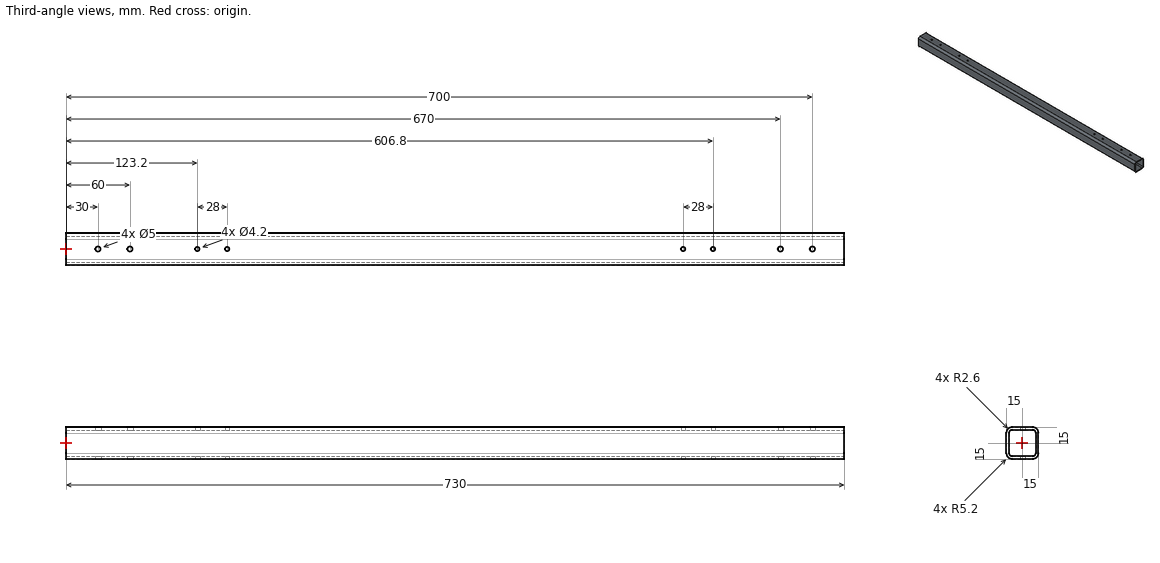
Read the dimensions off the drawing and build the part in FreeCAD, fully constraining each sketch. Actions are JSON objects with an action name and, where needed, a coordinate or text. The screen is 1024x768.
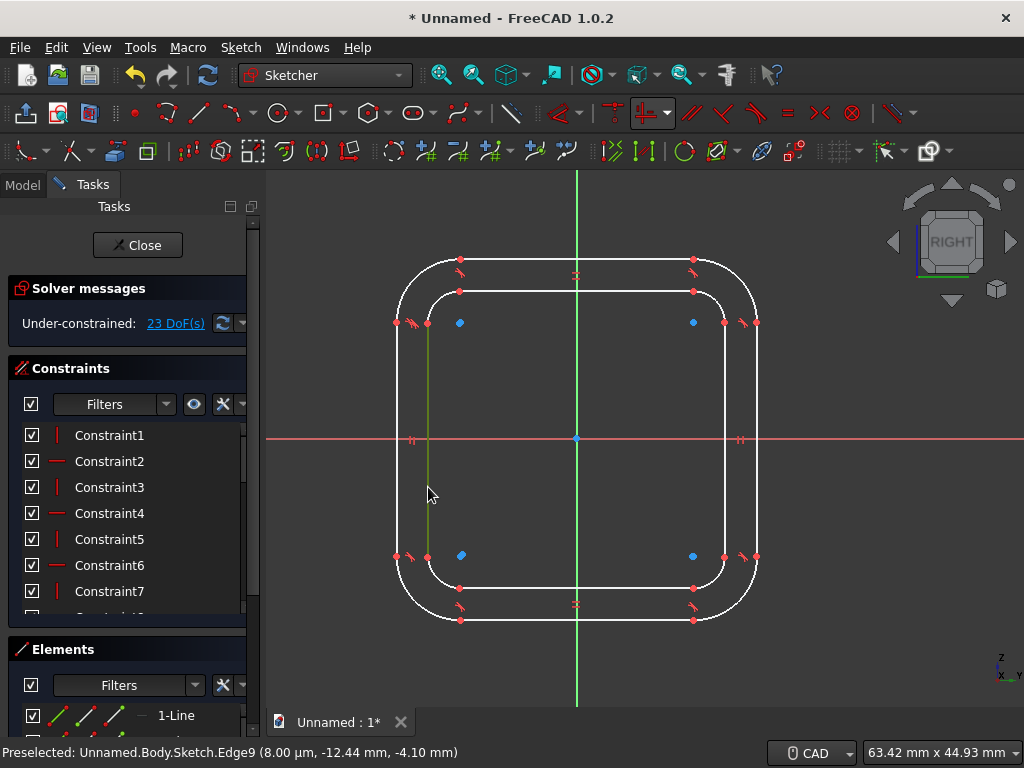
{"action": "left_click", "coordinate": [432, 571]}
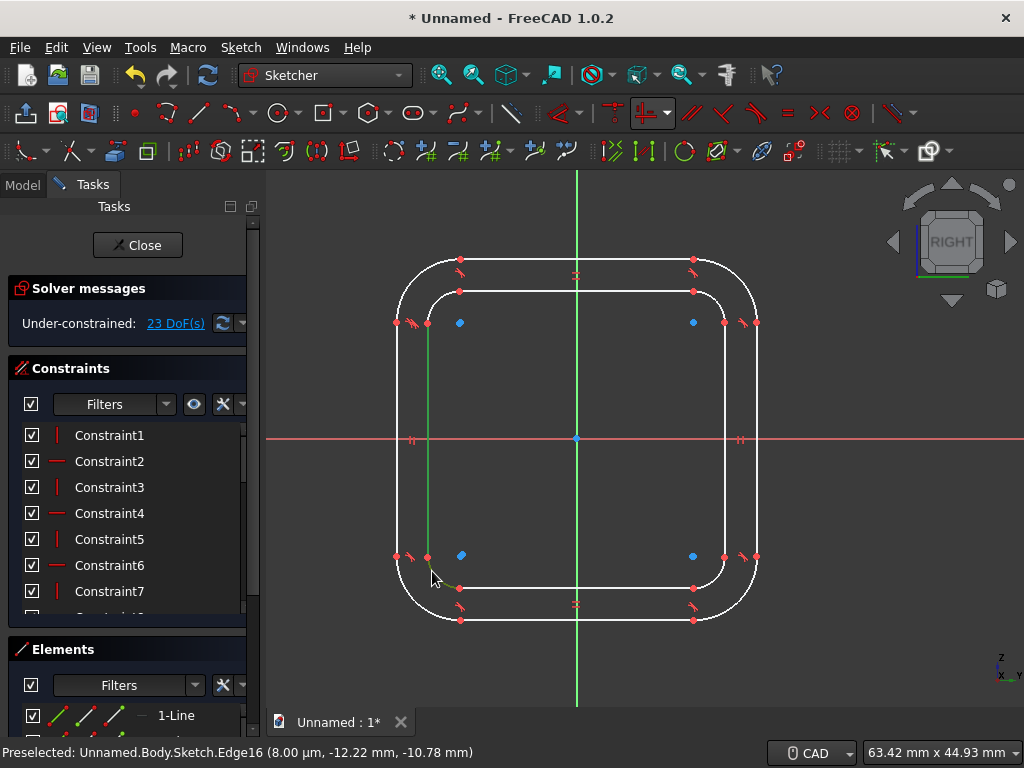
{"action": "left_click", "coordinate": [756, 114]}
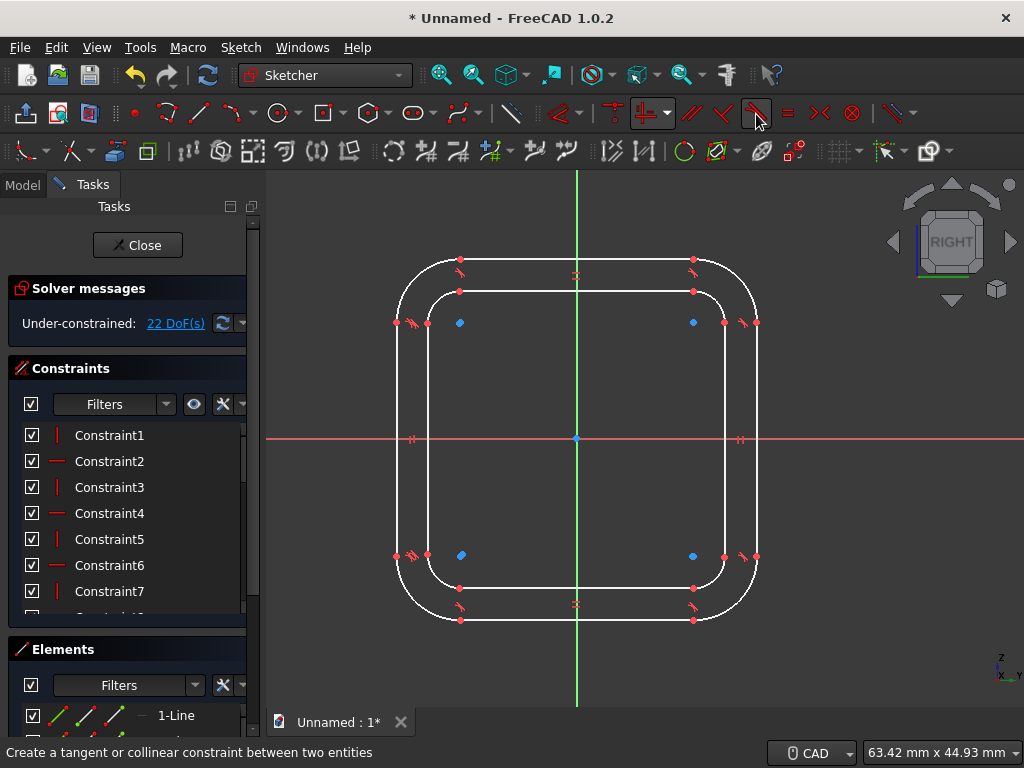
{"action": "left_click", "coordinate": [530, 291]}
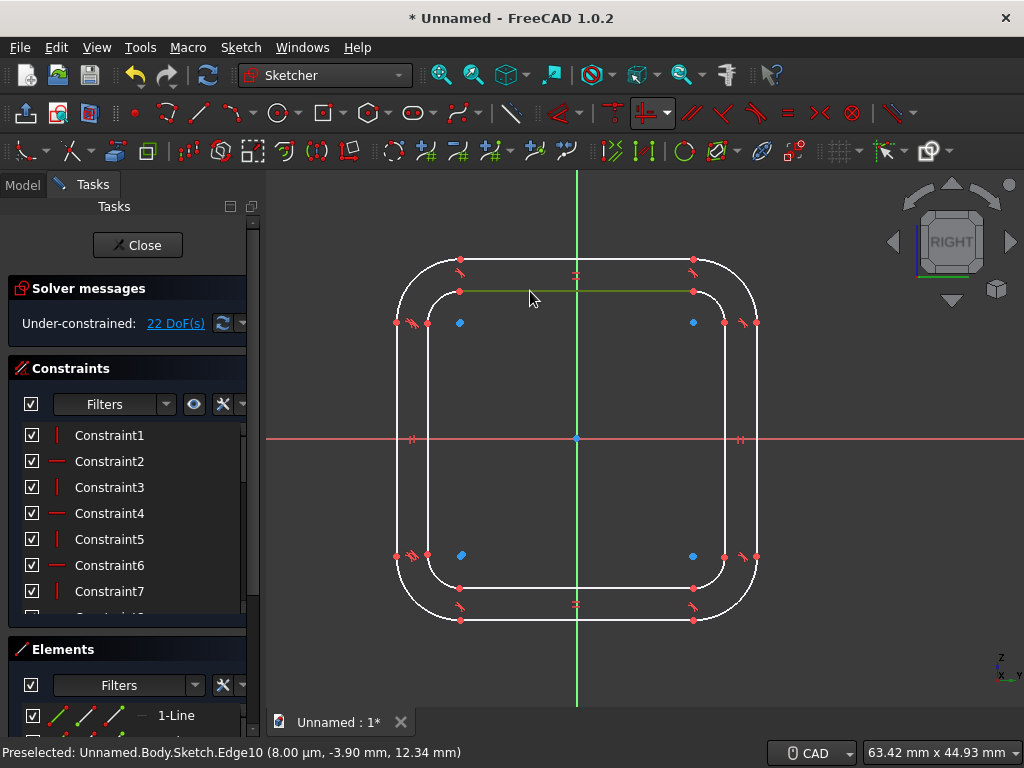
{"action": "left_click", "coordinate": [445, 295]}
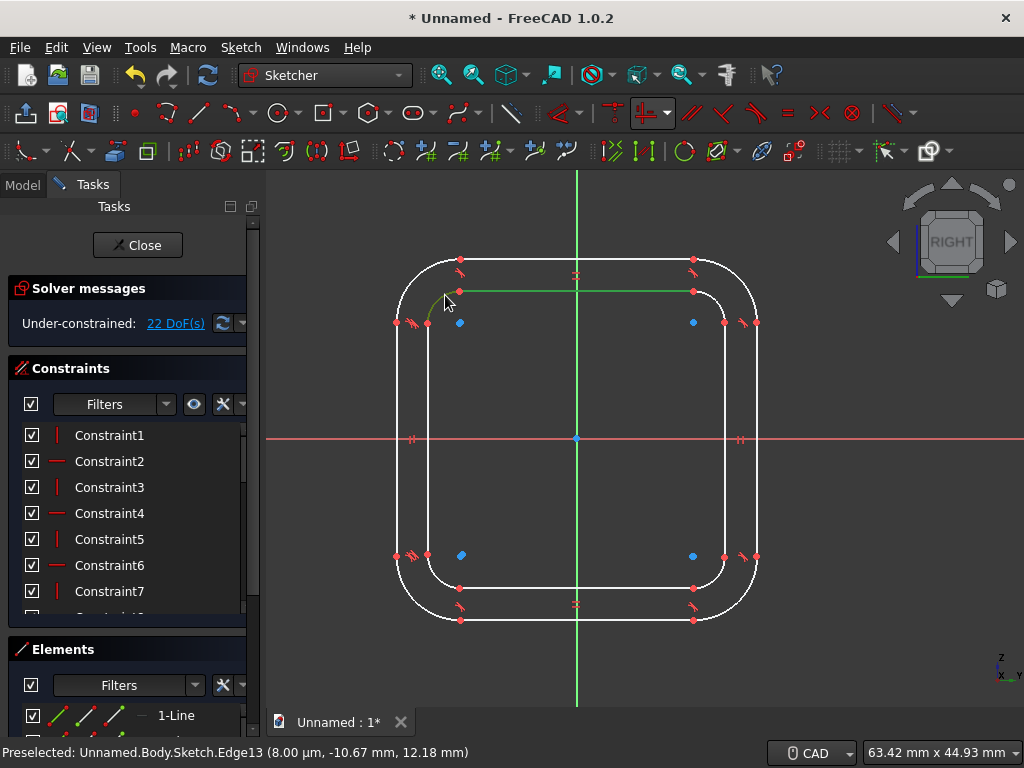
{"action": "left_click", "coordinate": [756, 114]}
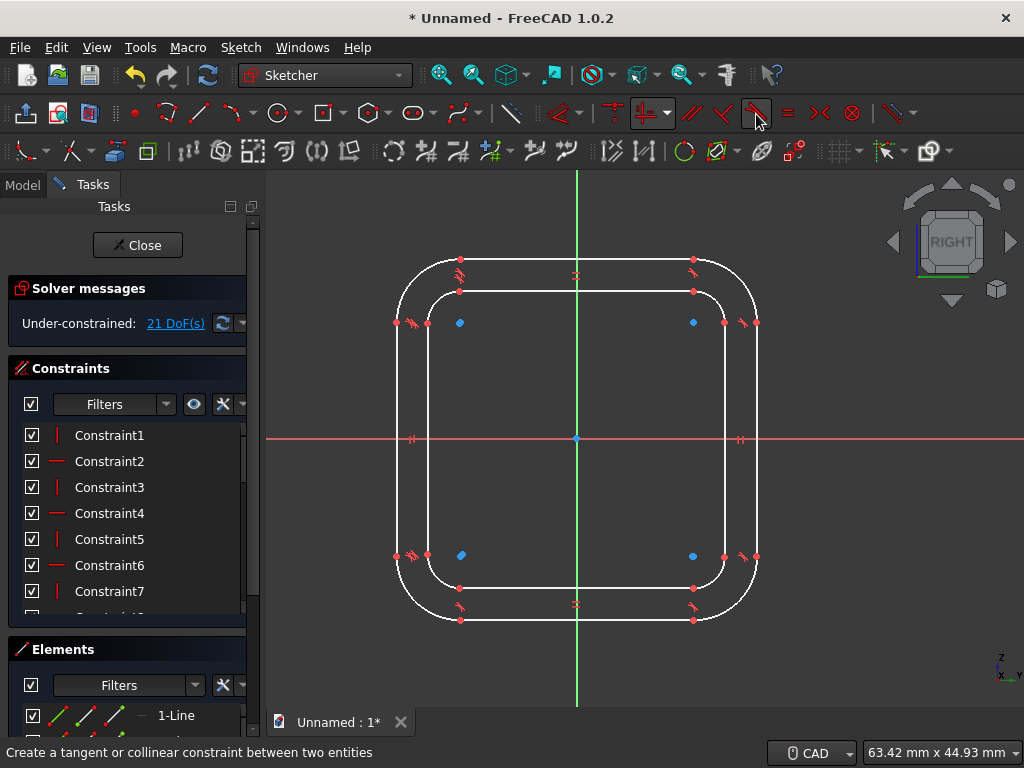
{"action": "left_click", "coordinate": [530, 291]}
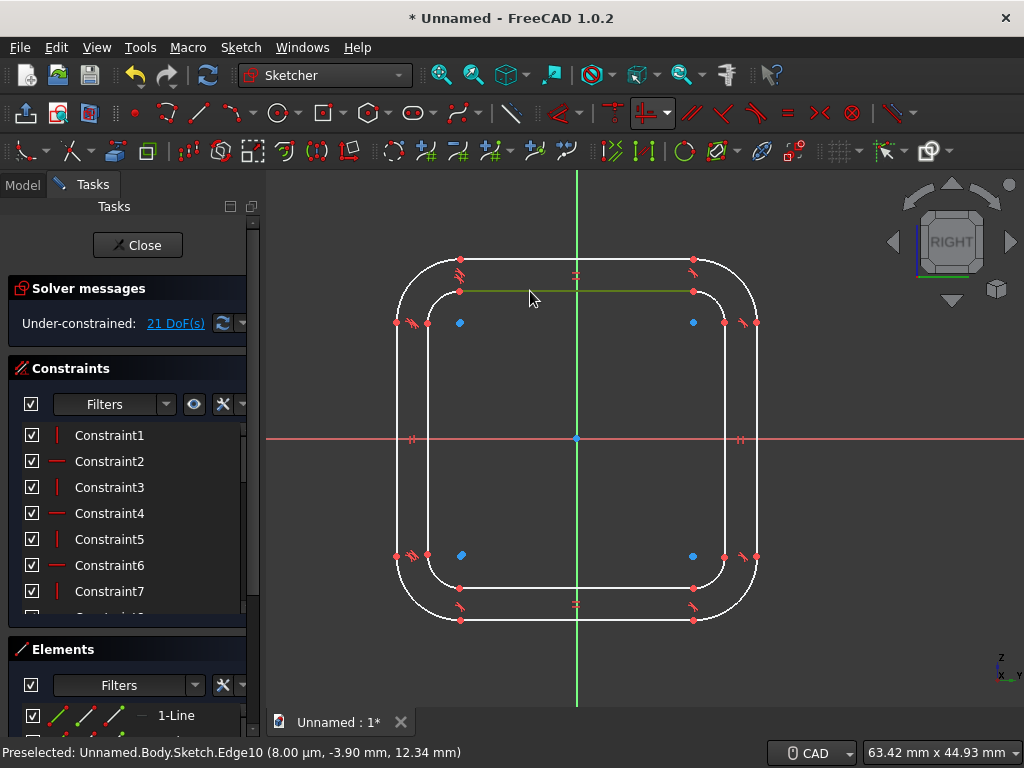
{"action": "left_click", "coordinate": [721, 308]}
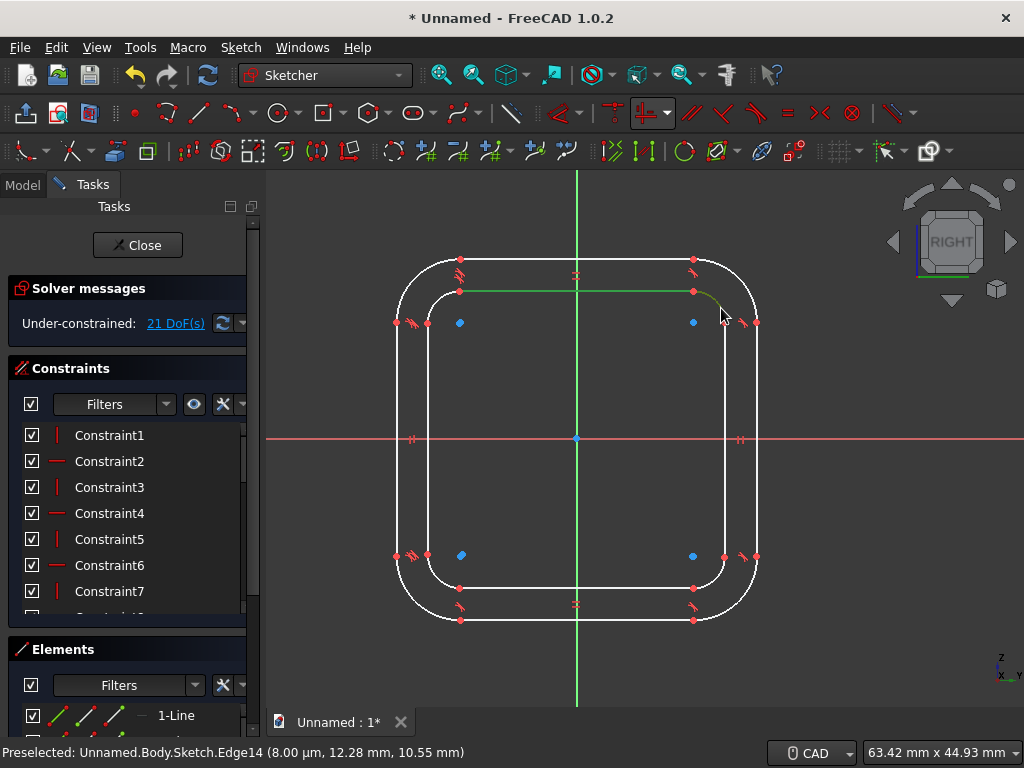
{"action": "left_click", "coordinate": [756, 114]}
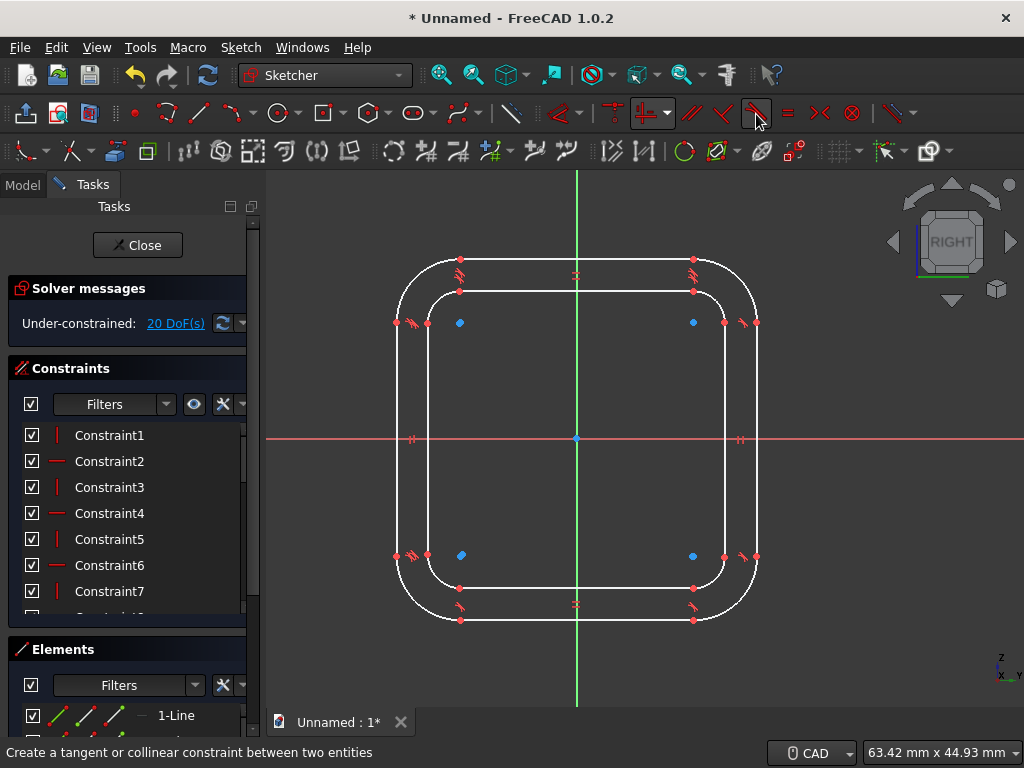
{"action": "left_click", "coordinate": [725, 393]}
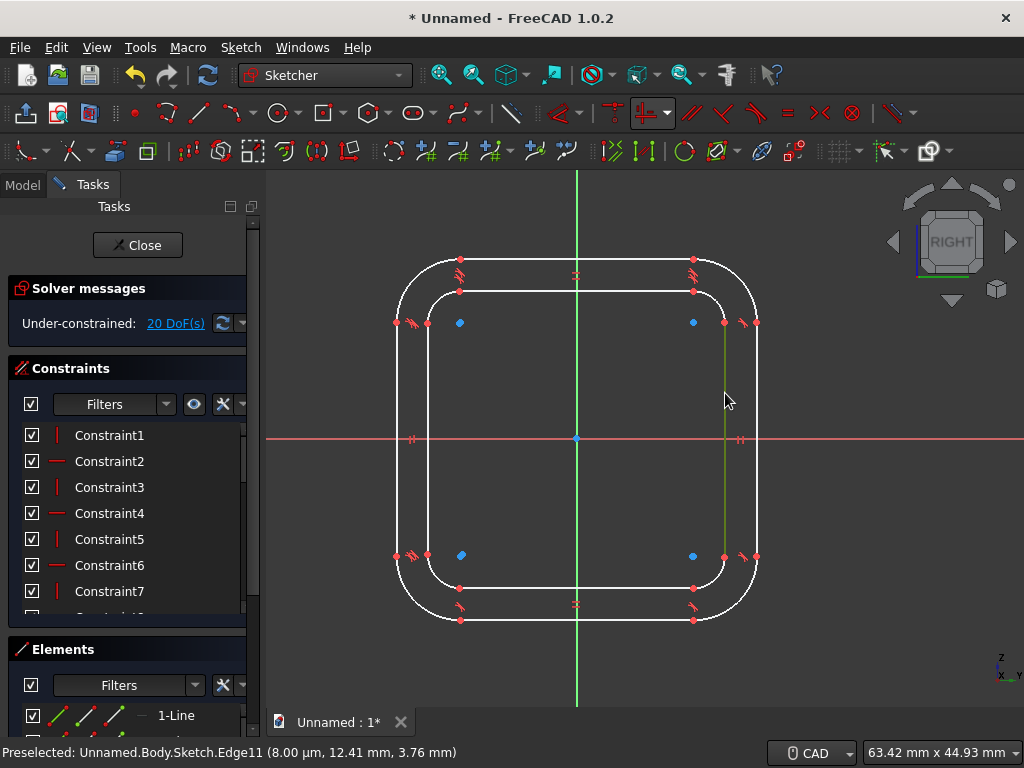
{"action": "left_click", "coordinate": [721, 308]}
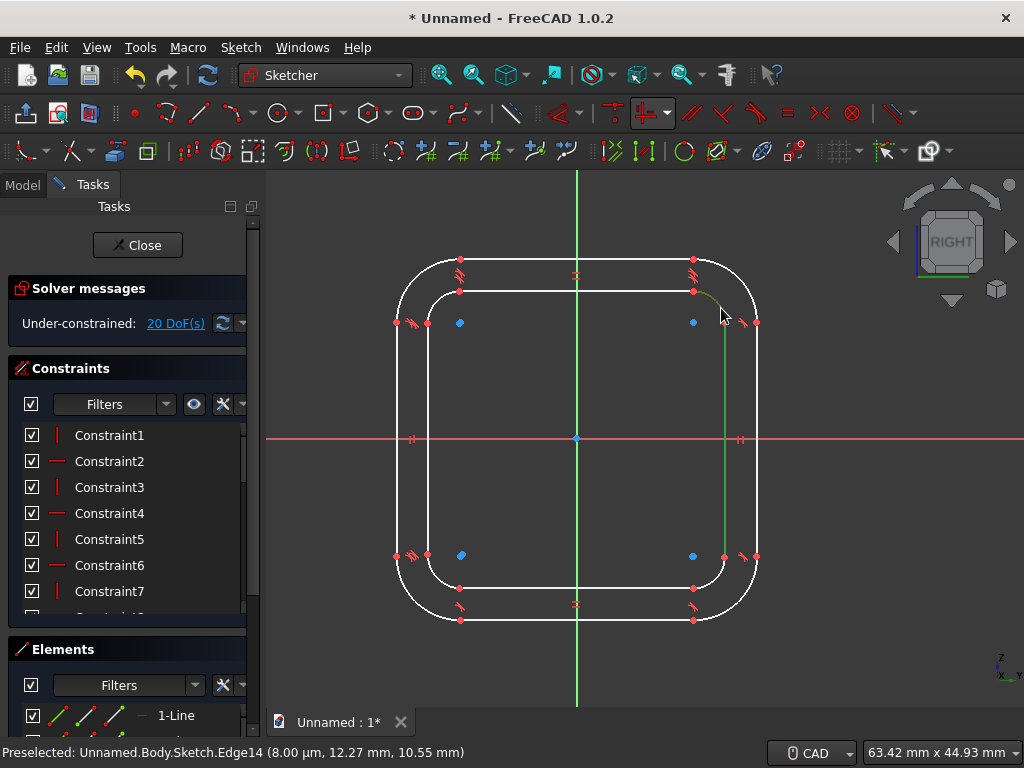
{"action": "left_click", "coordinate": [756, 114]}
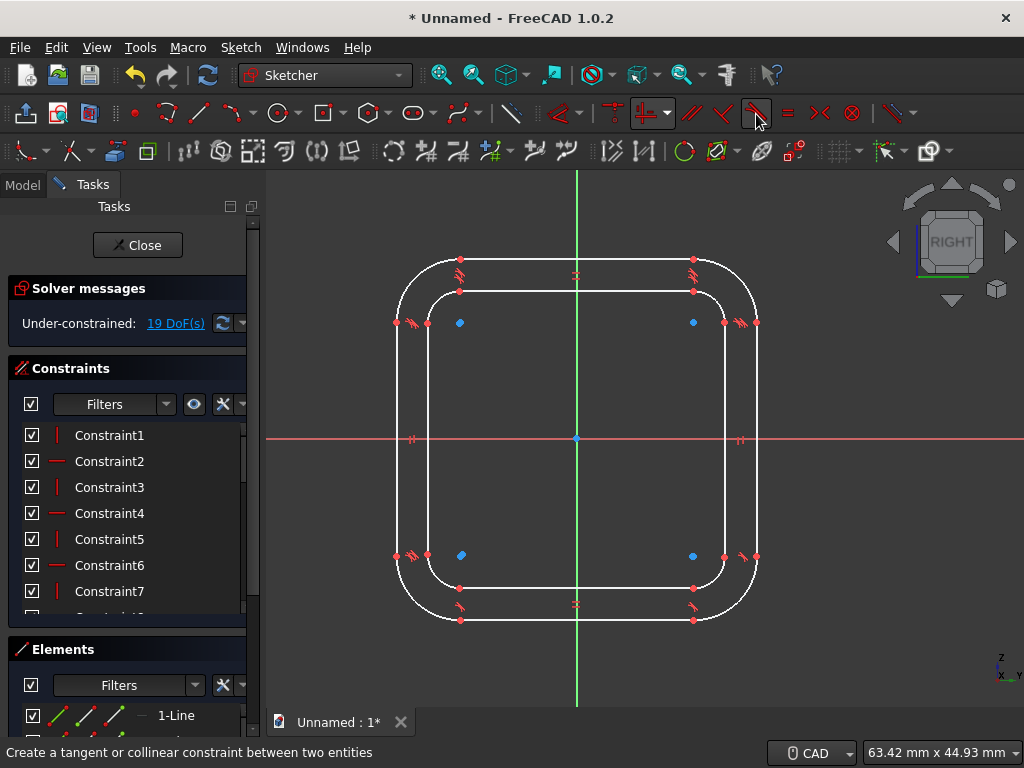
{"action": "left_click", "coordinate": [725, 393]}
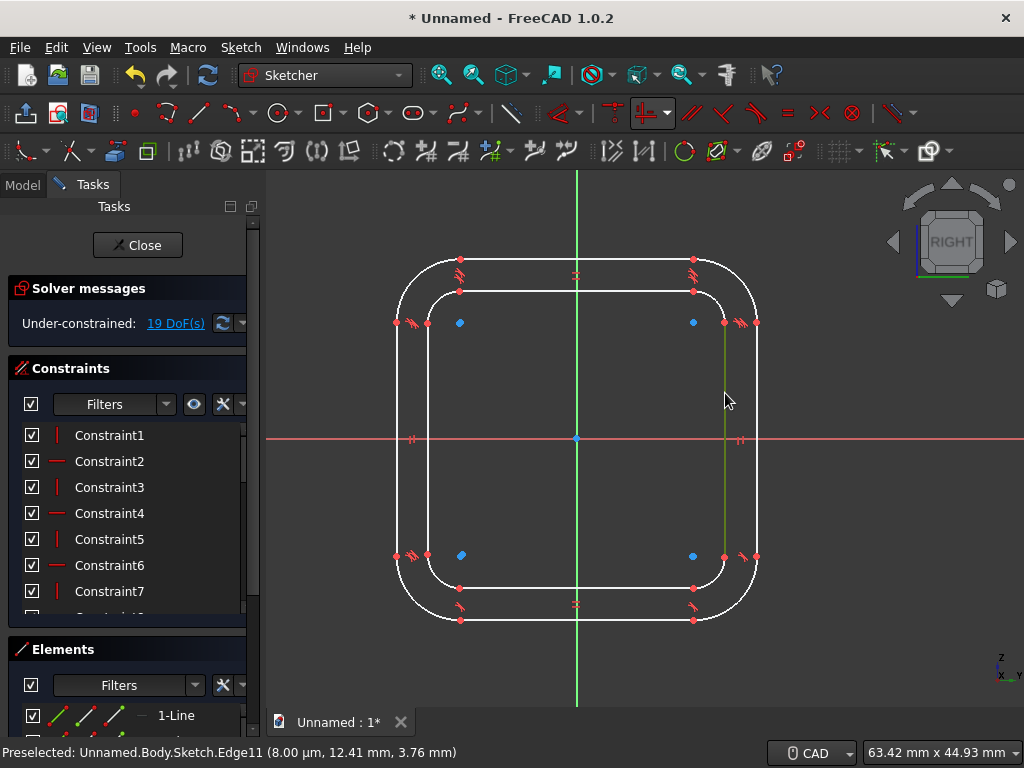
{"action": "left_click", "coordinate": [708, 585]}